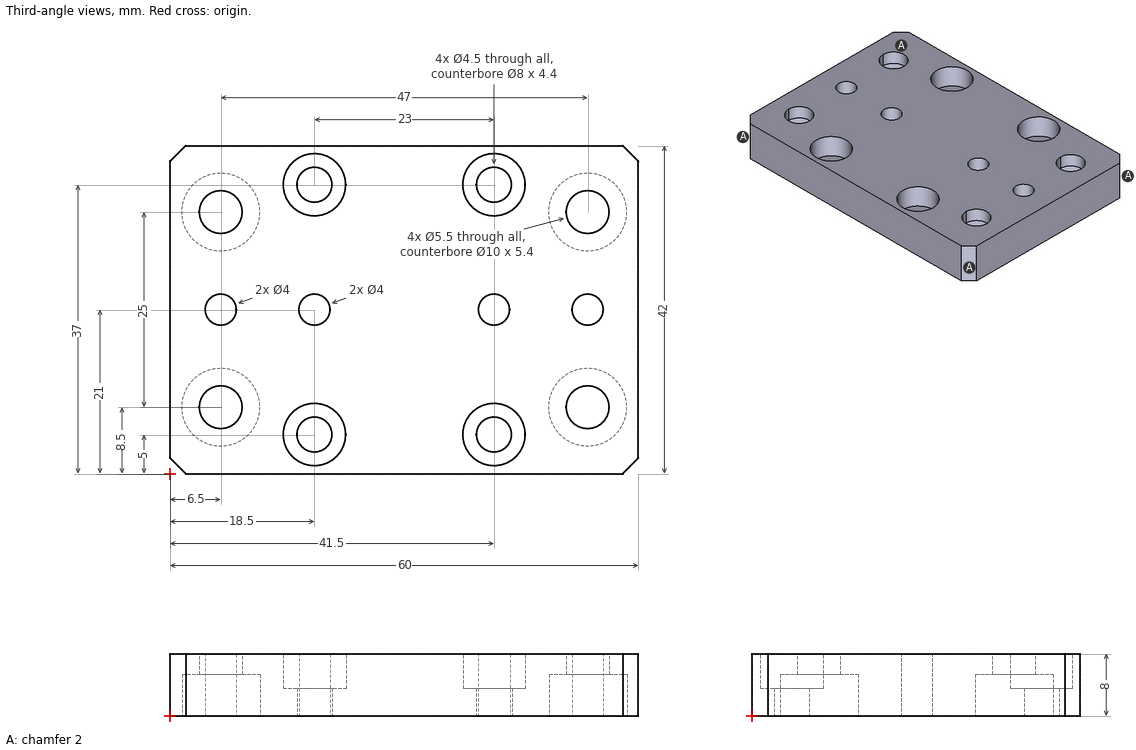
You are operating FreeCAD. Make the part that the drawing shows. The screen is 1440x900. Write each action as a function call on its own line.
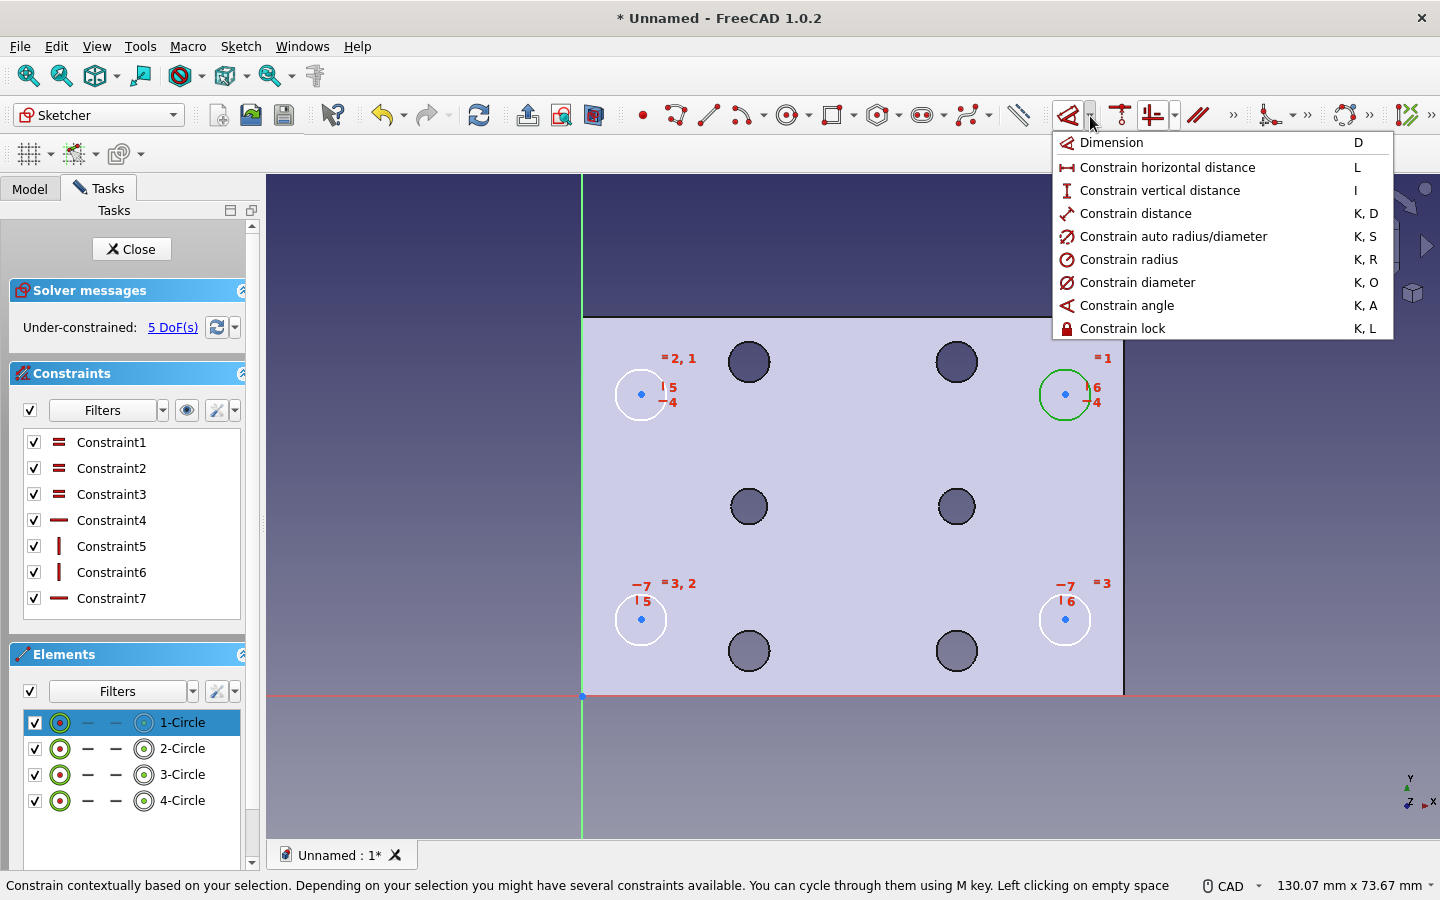
click(1223, 282)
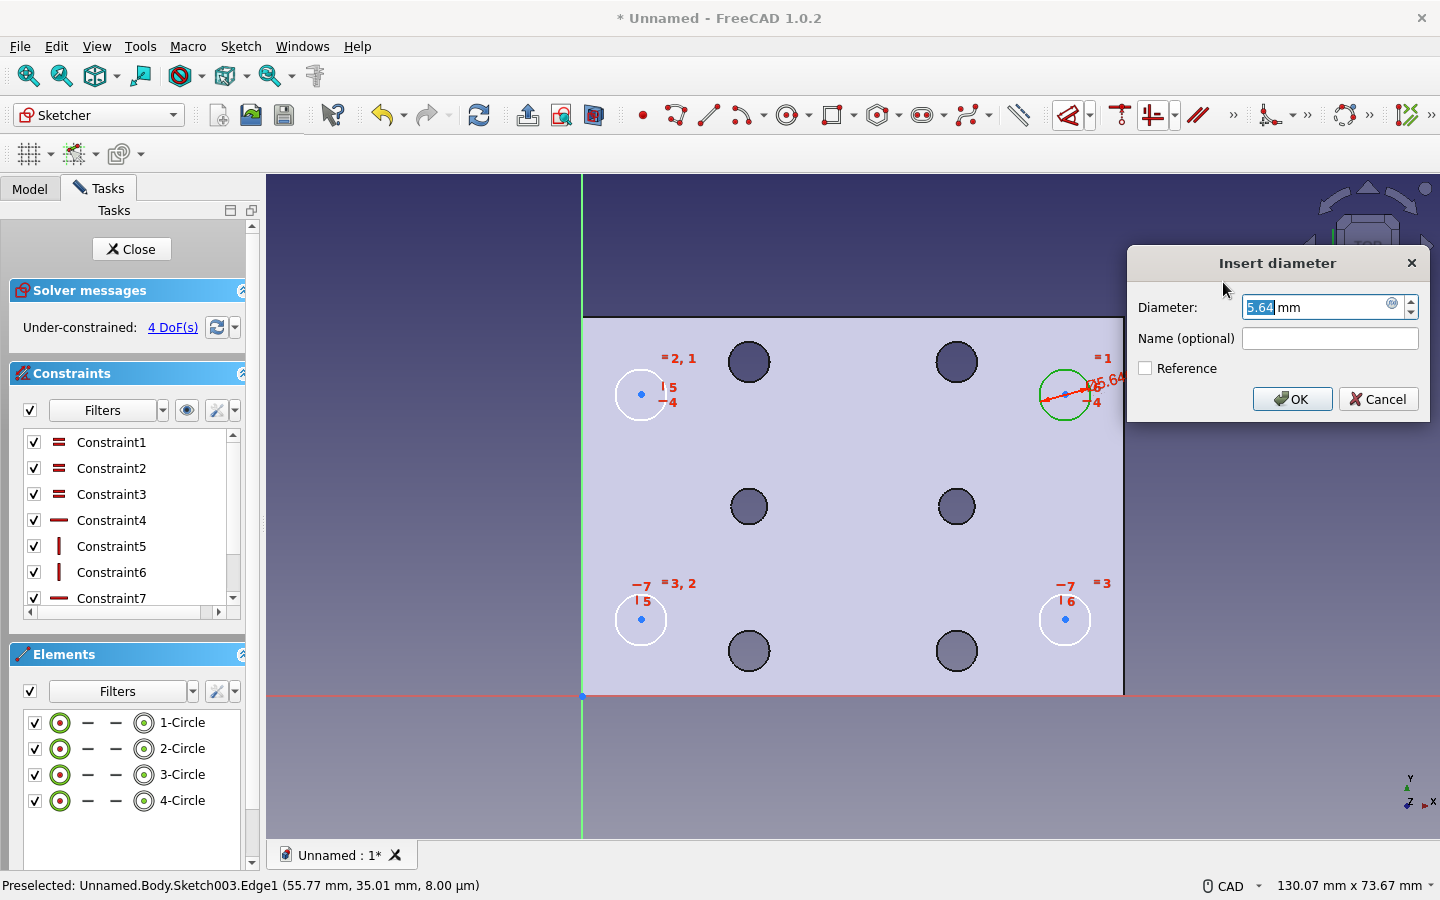
text(5.5)
key(Return)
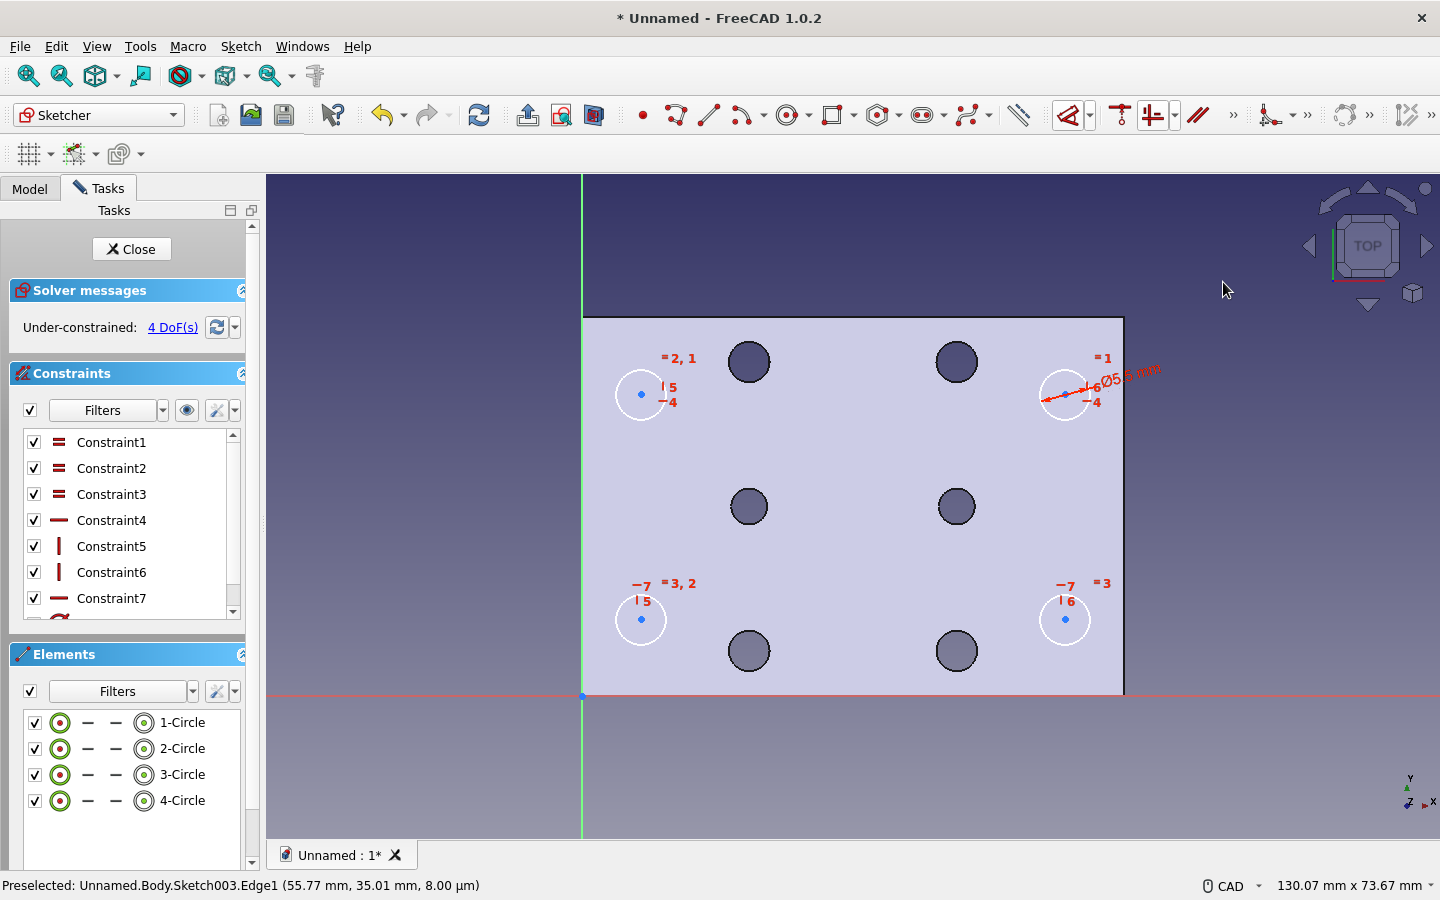
click(641, 395)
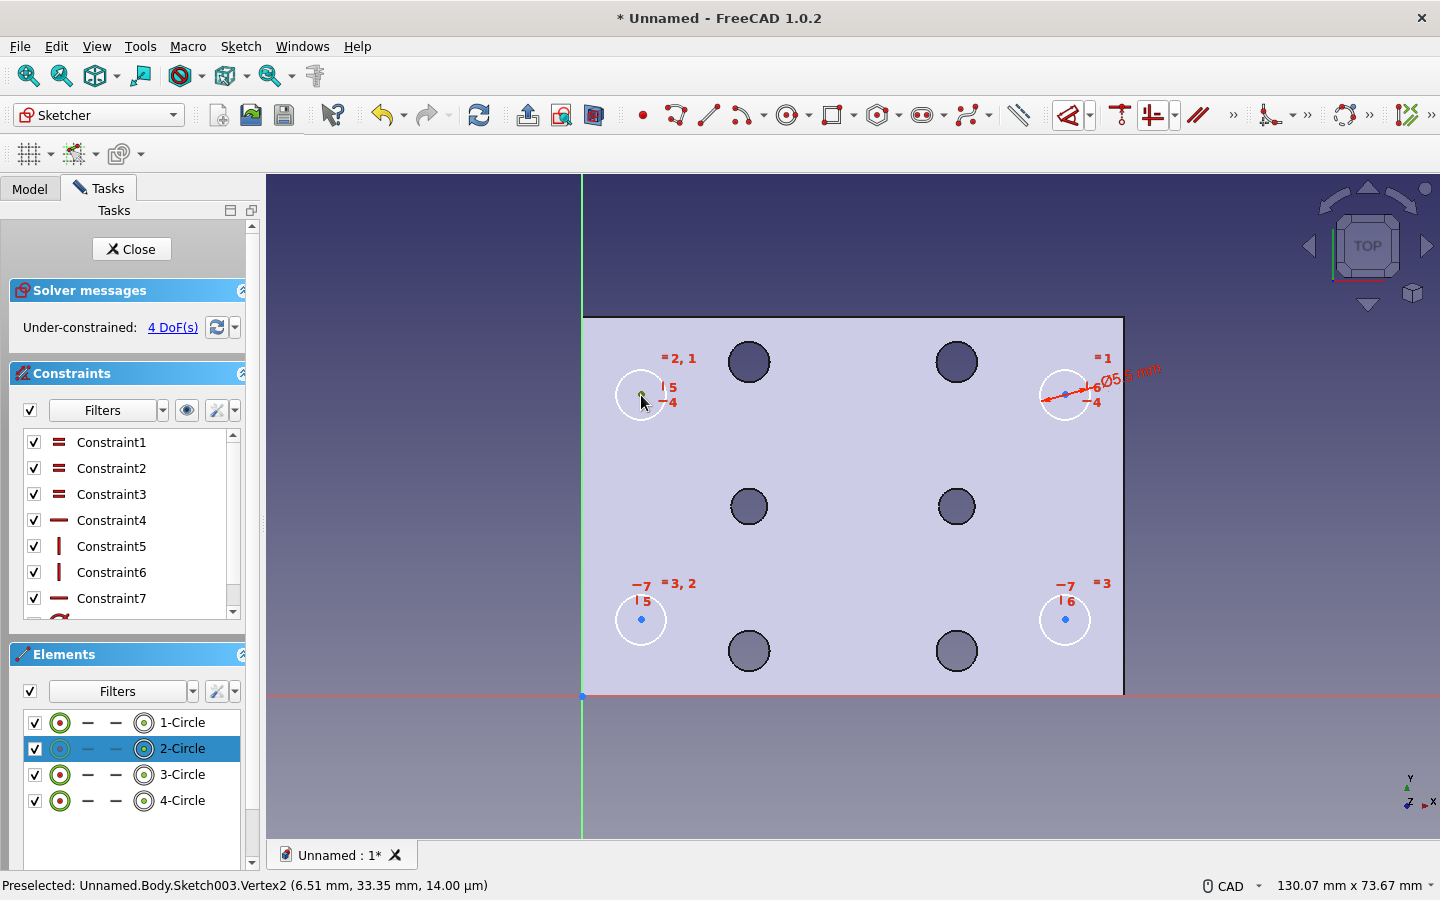
click(1090, 116)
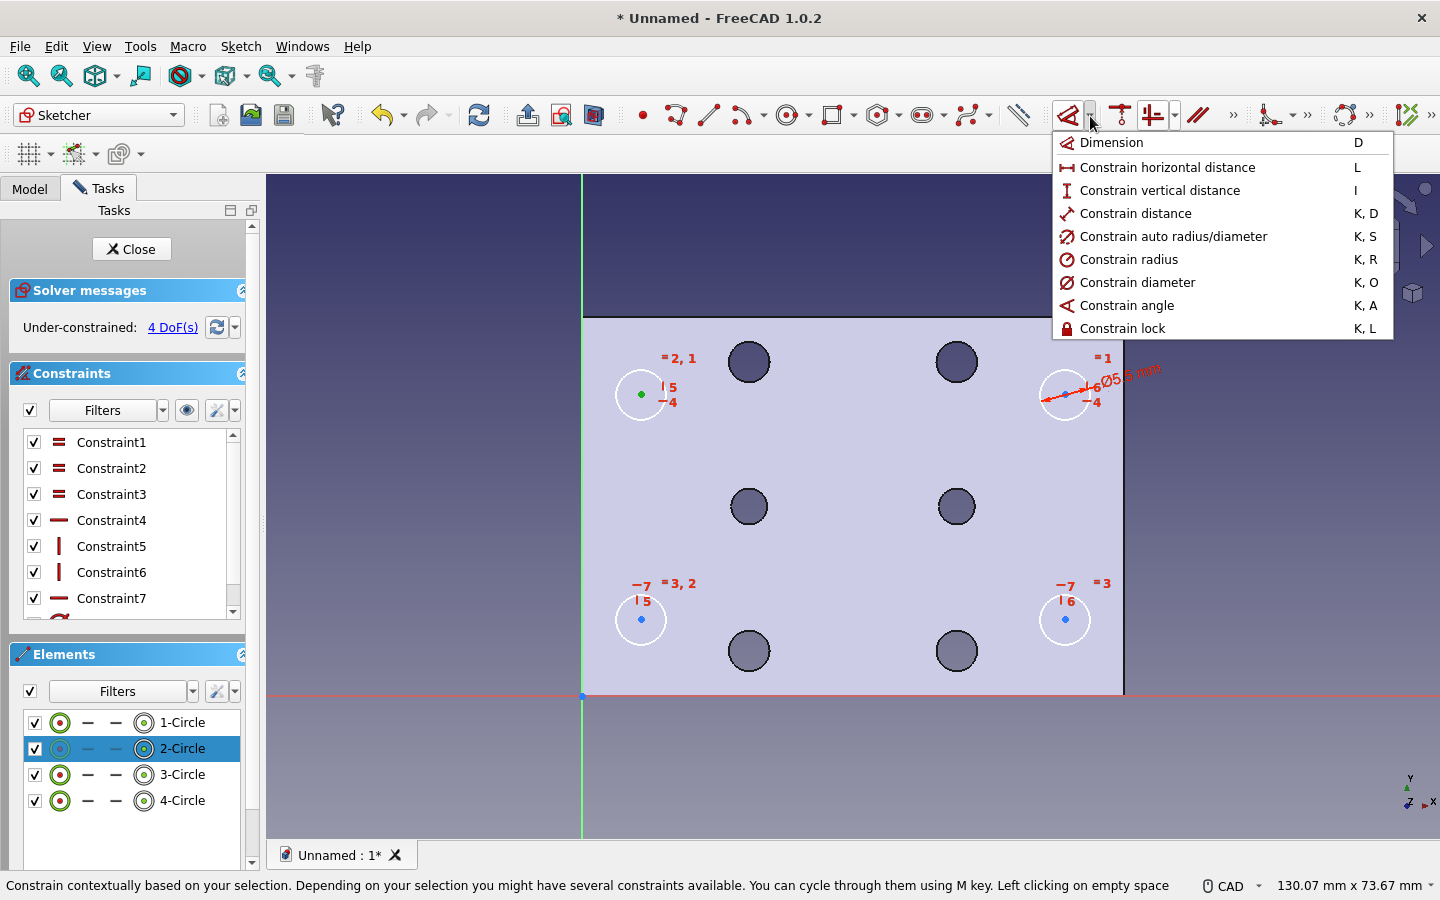
click(1223, 168)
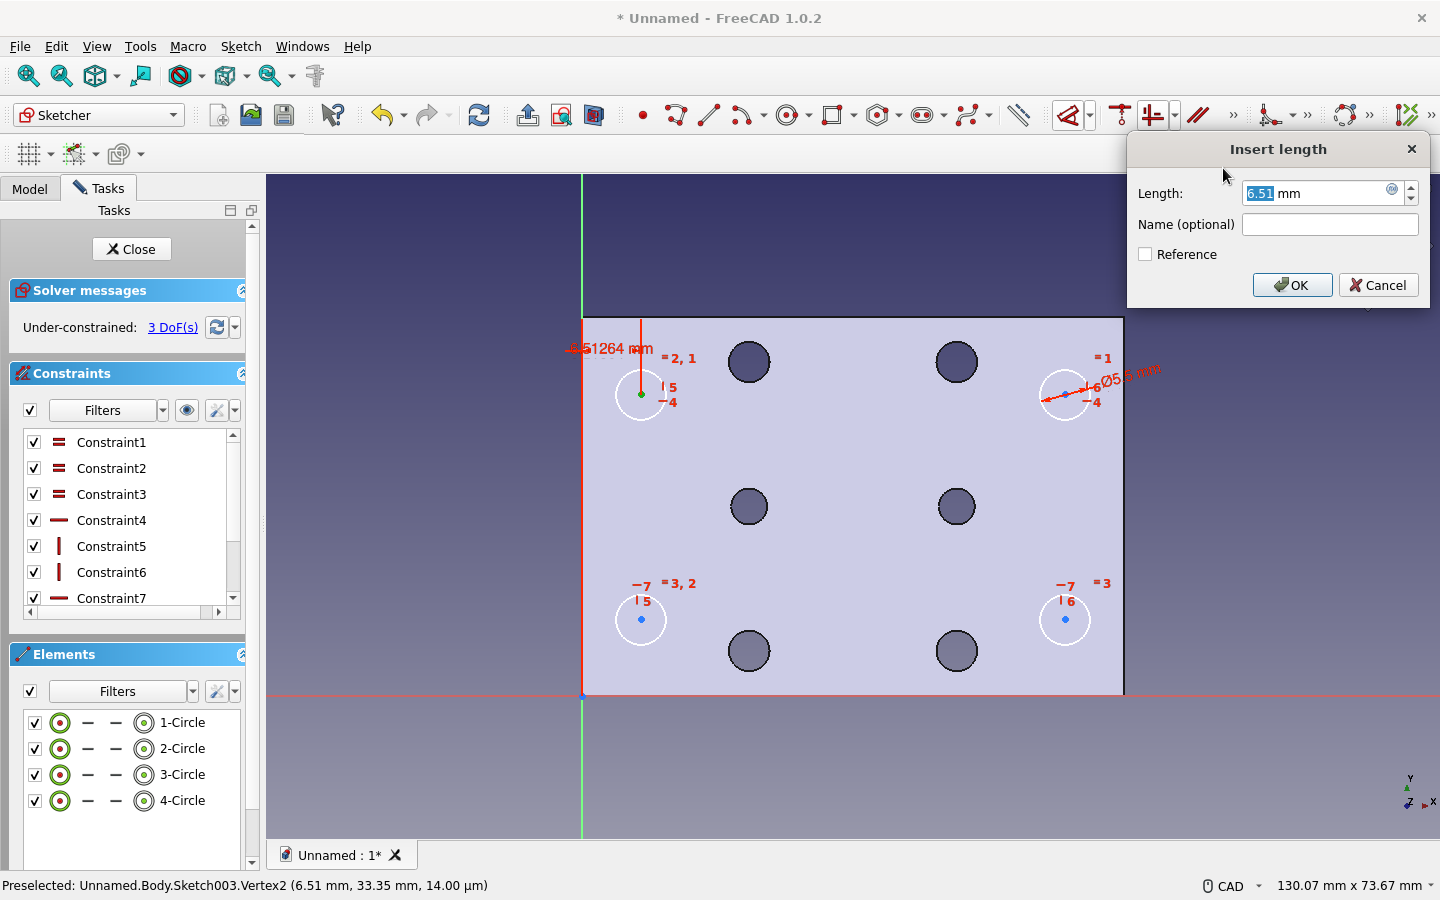
text(6.5)
key(Return)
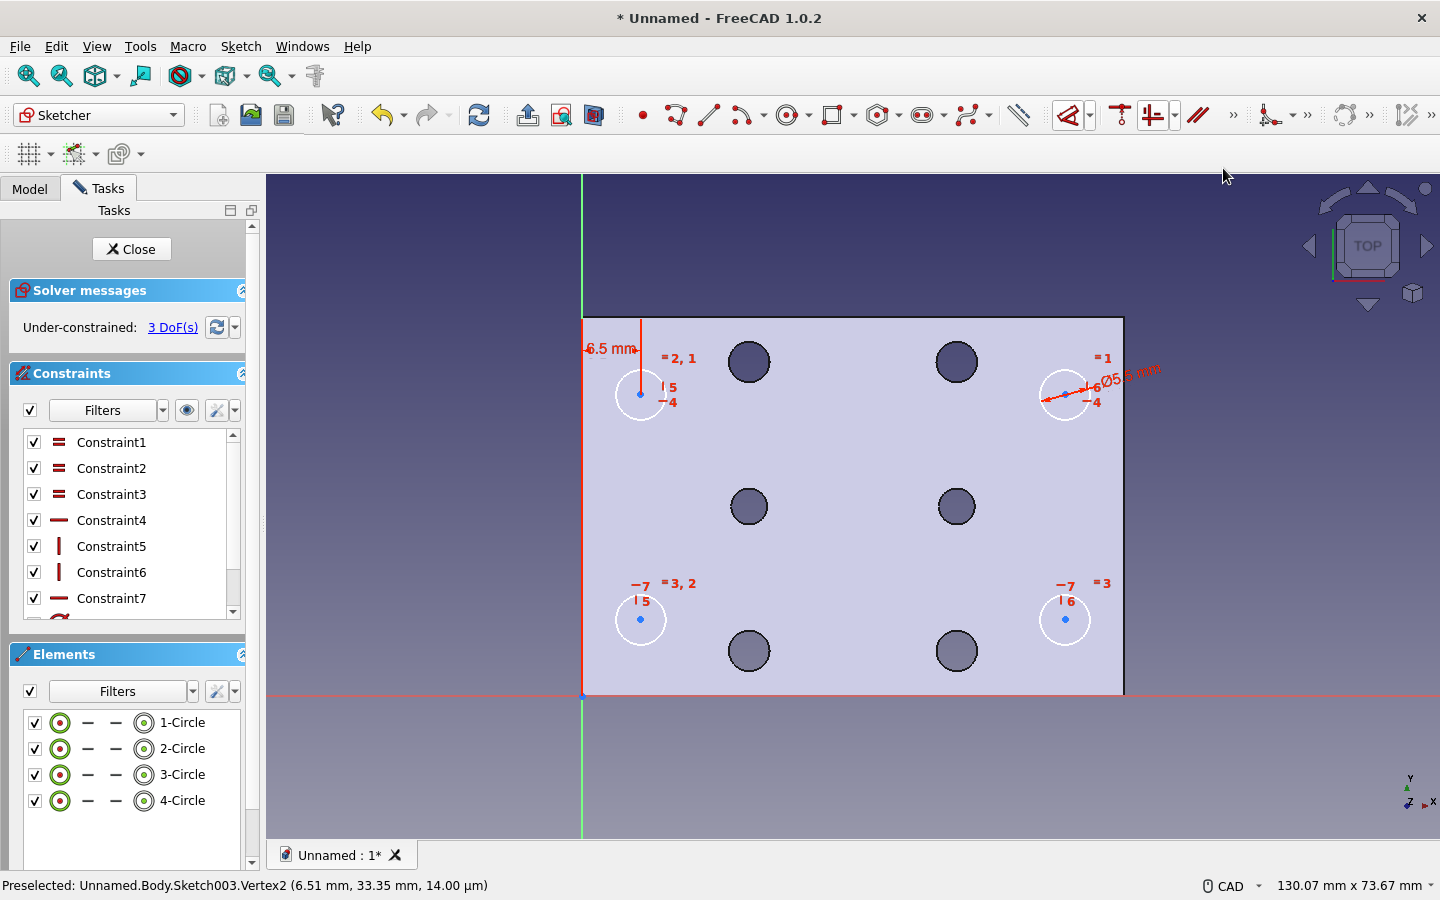
click(641, 620)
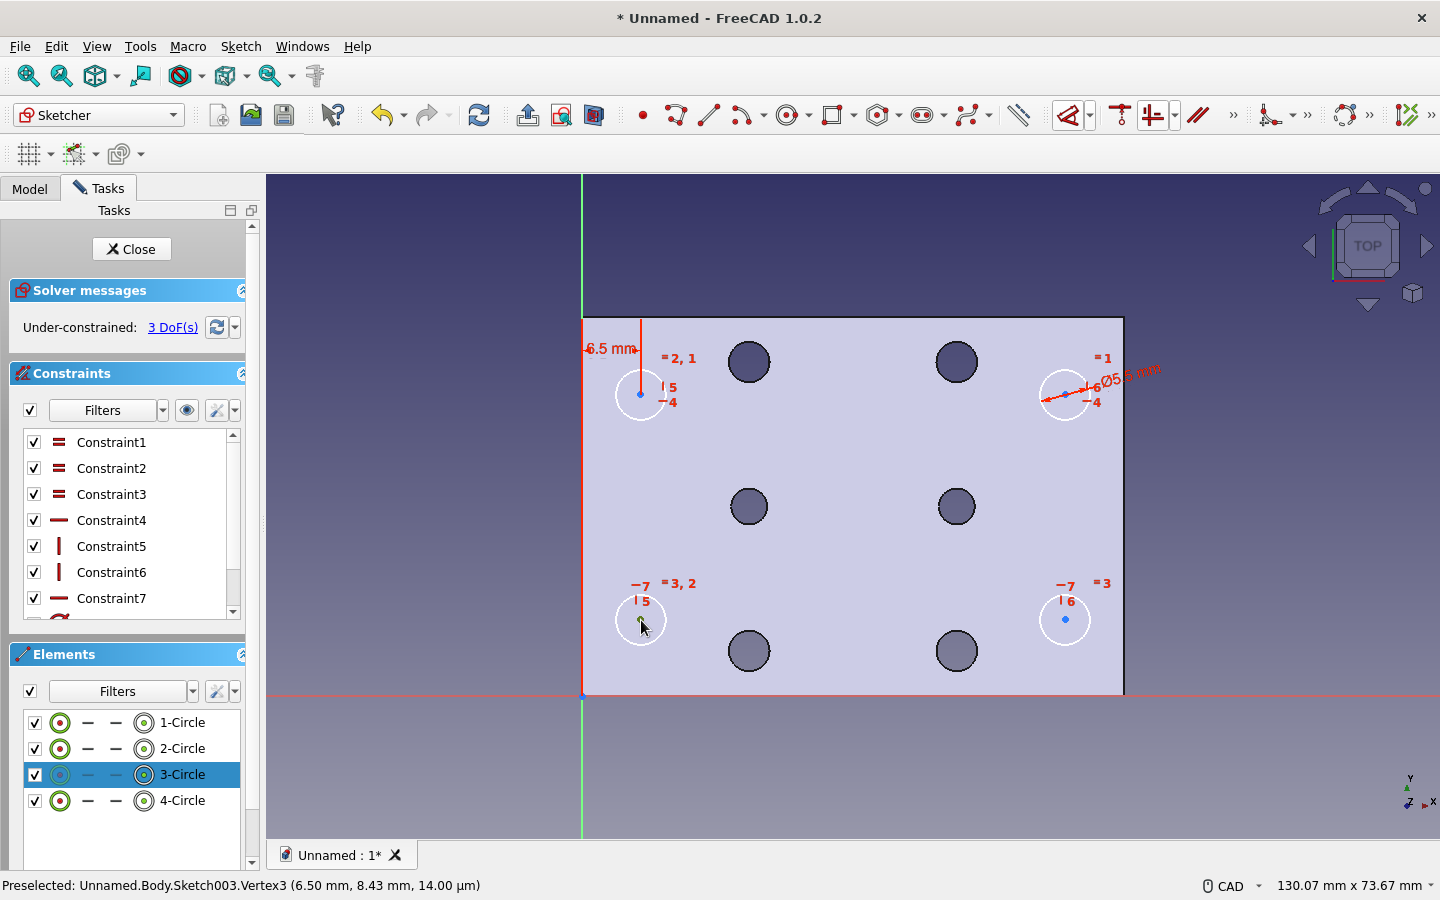
click(1090, 116)